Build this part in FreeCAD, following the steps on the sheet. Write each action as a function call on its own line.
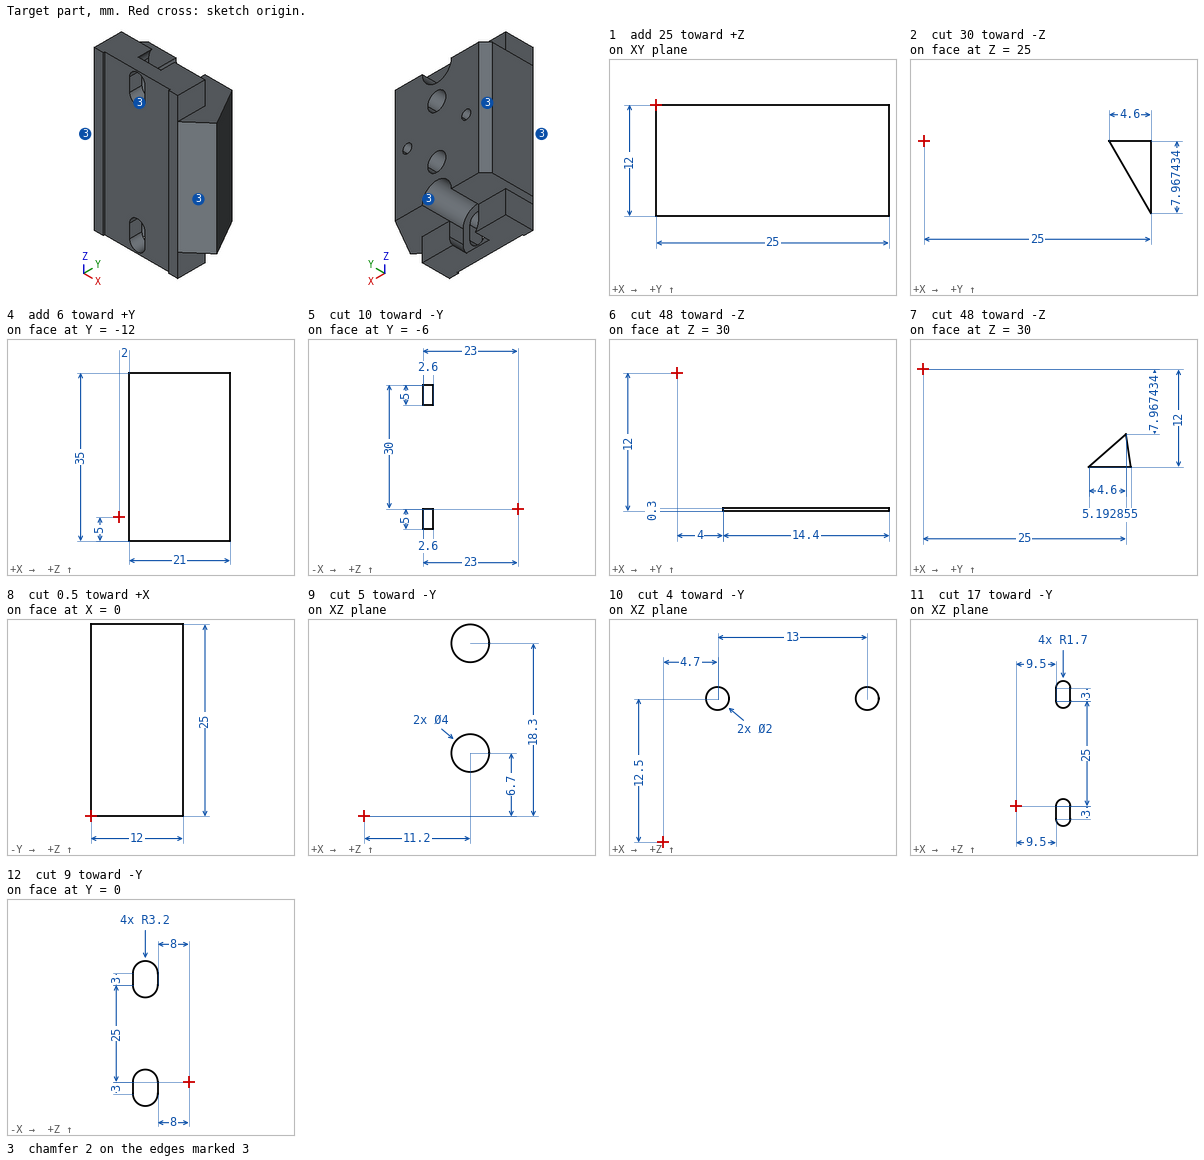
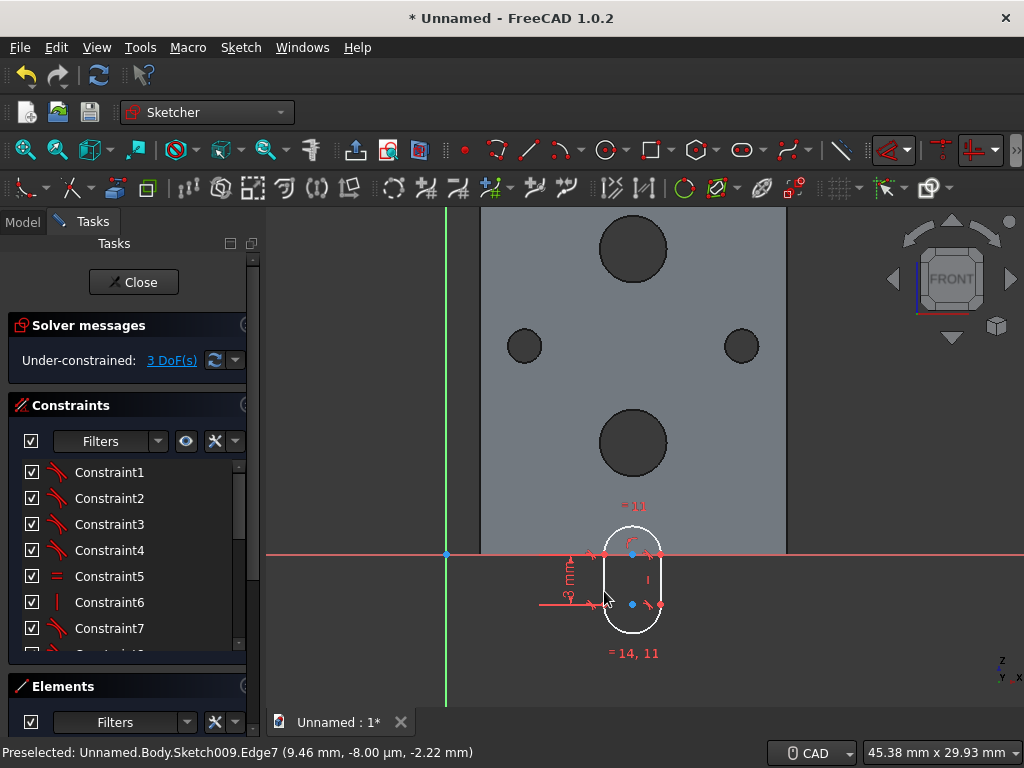
scroll(604, 592, down, 3)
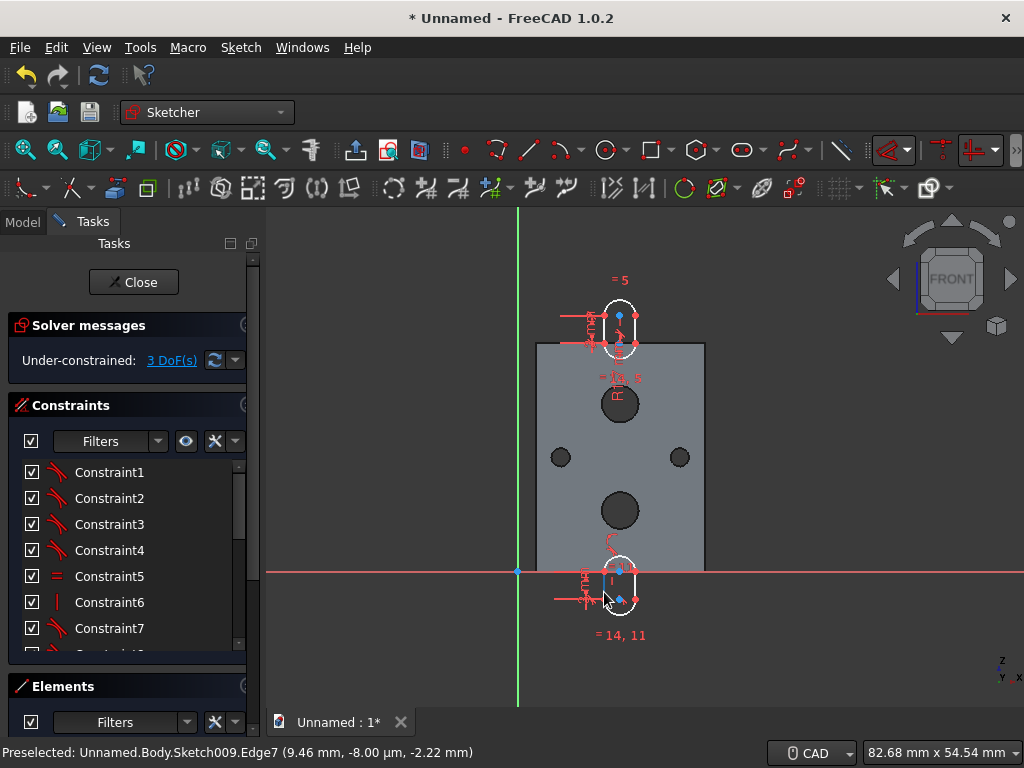
click(604, 343)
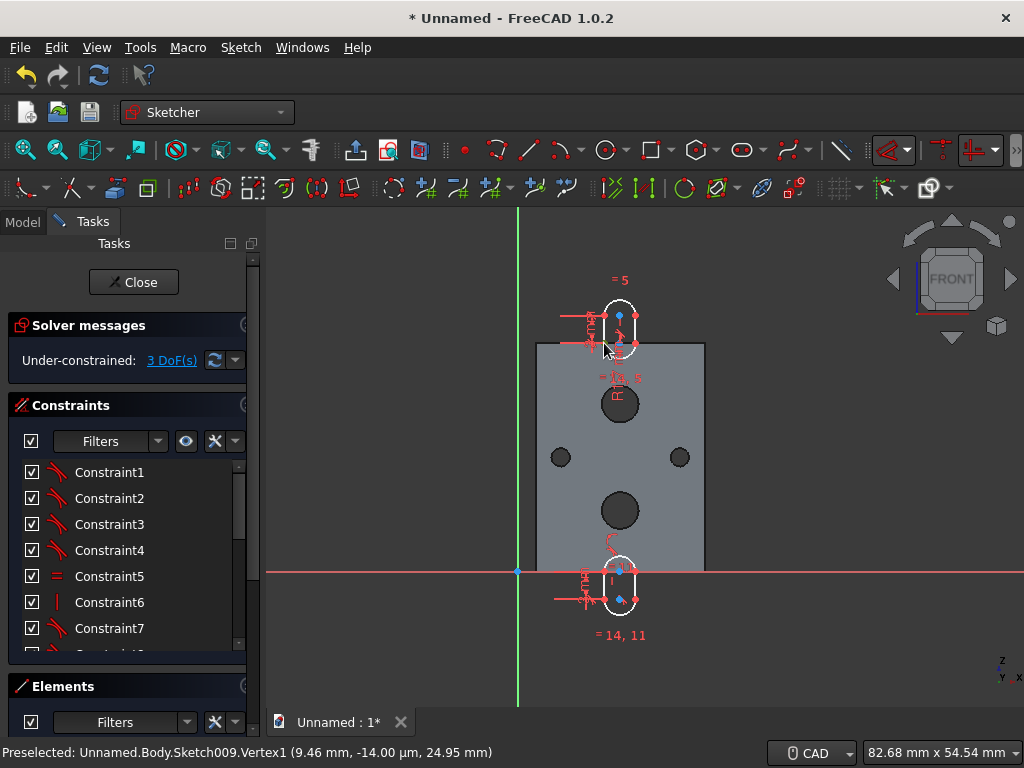
key(i)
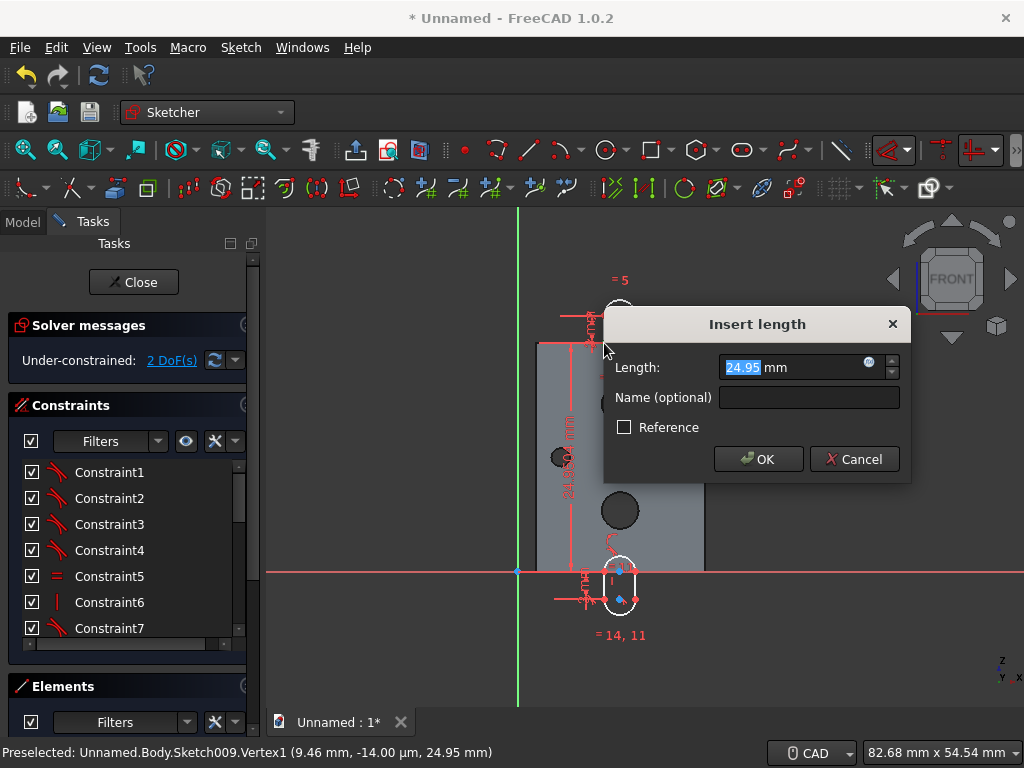
text(25)
key(Return)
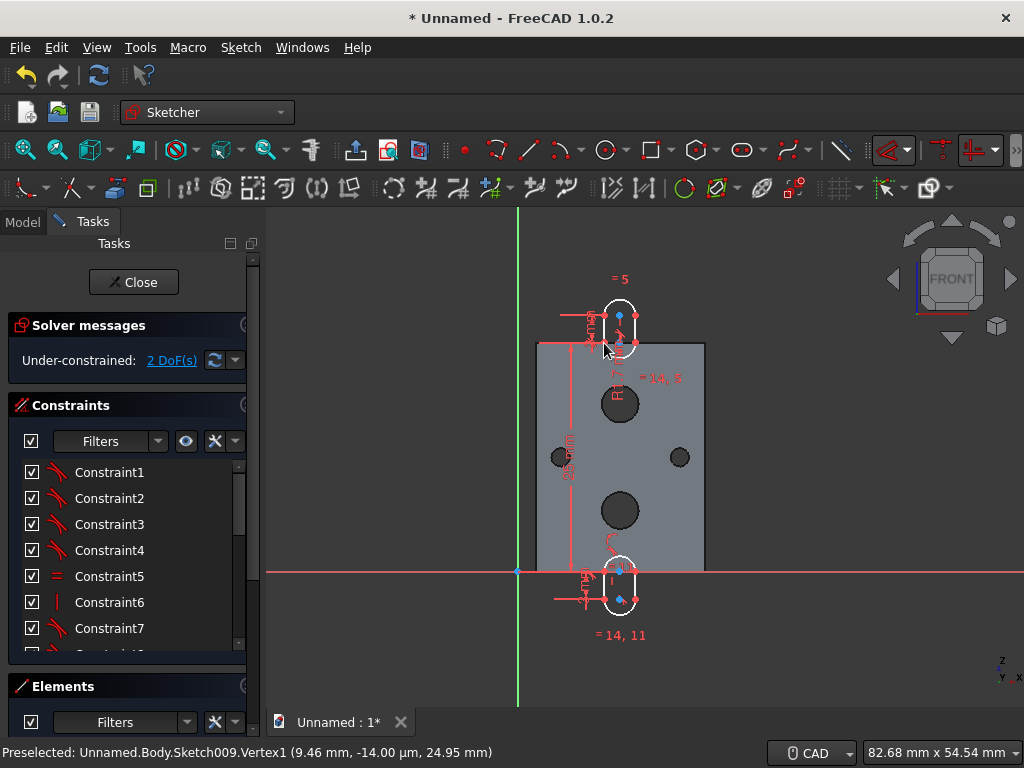
click(604, 343)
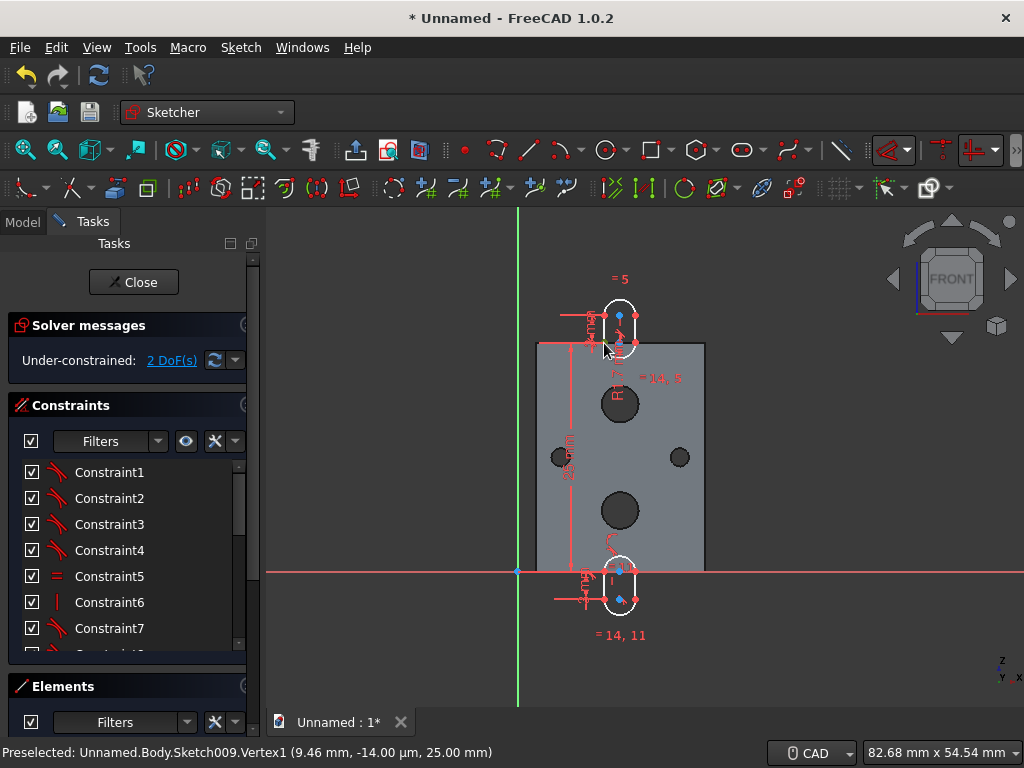
key(l)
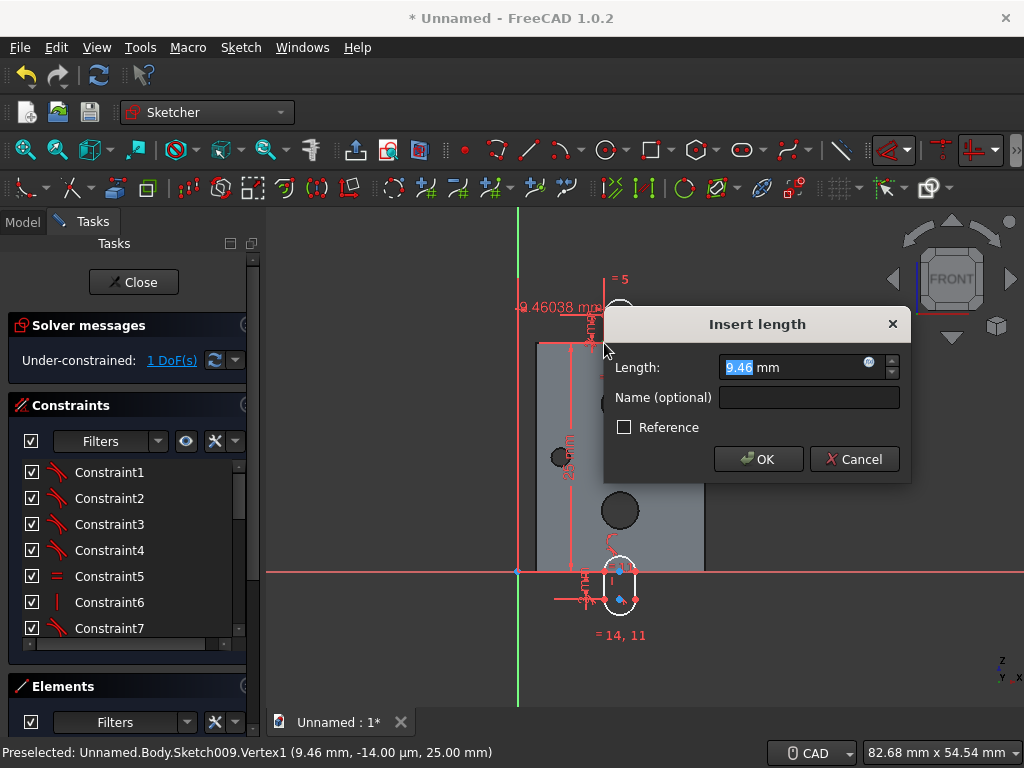
text(9.5)
key(Return)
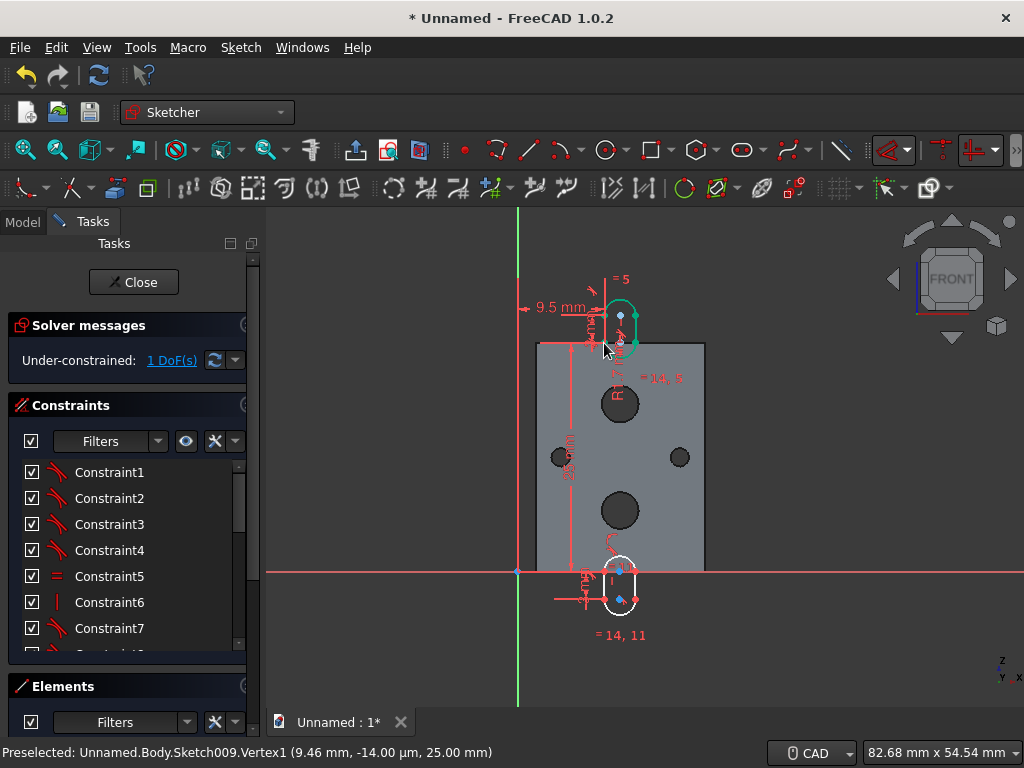
click(604, 599)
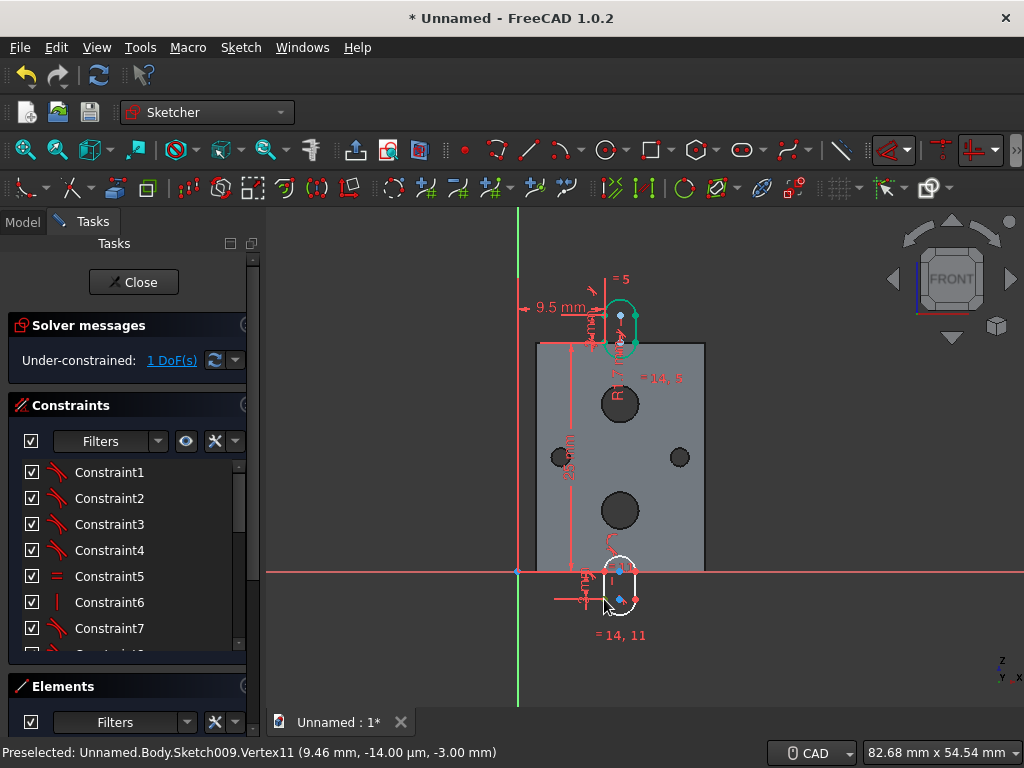
key(l)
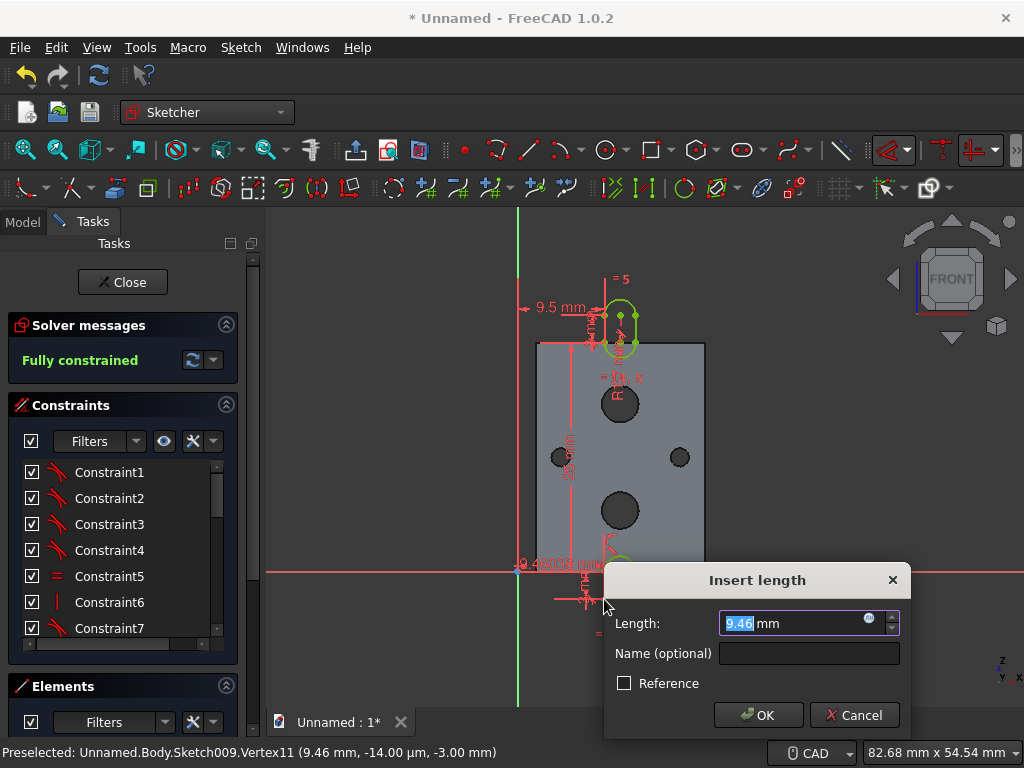
text(9.5)
key(Return)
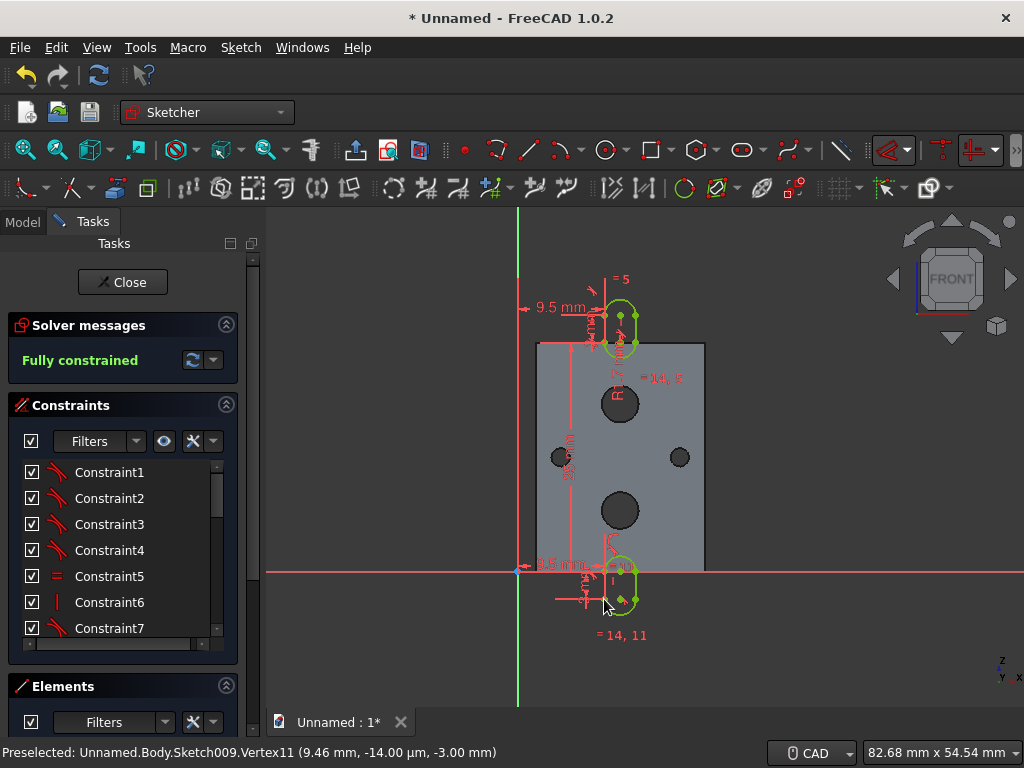
click(123, 282)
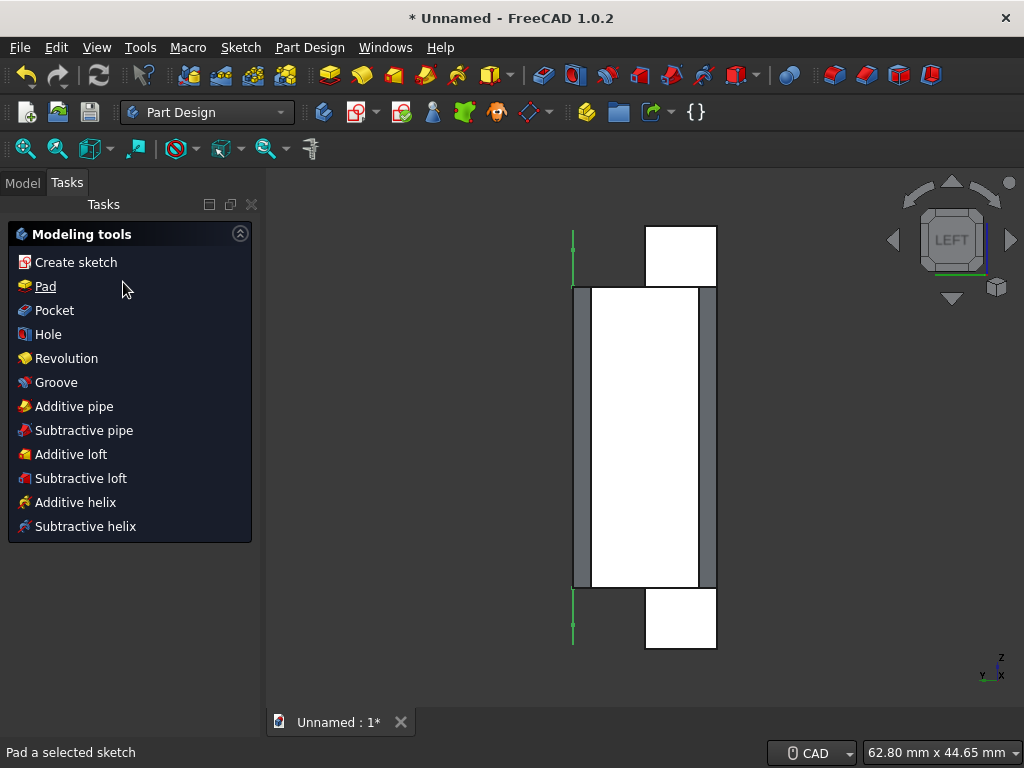
click(544, 76)